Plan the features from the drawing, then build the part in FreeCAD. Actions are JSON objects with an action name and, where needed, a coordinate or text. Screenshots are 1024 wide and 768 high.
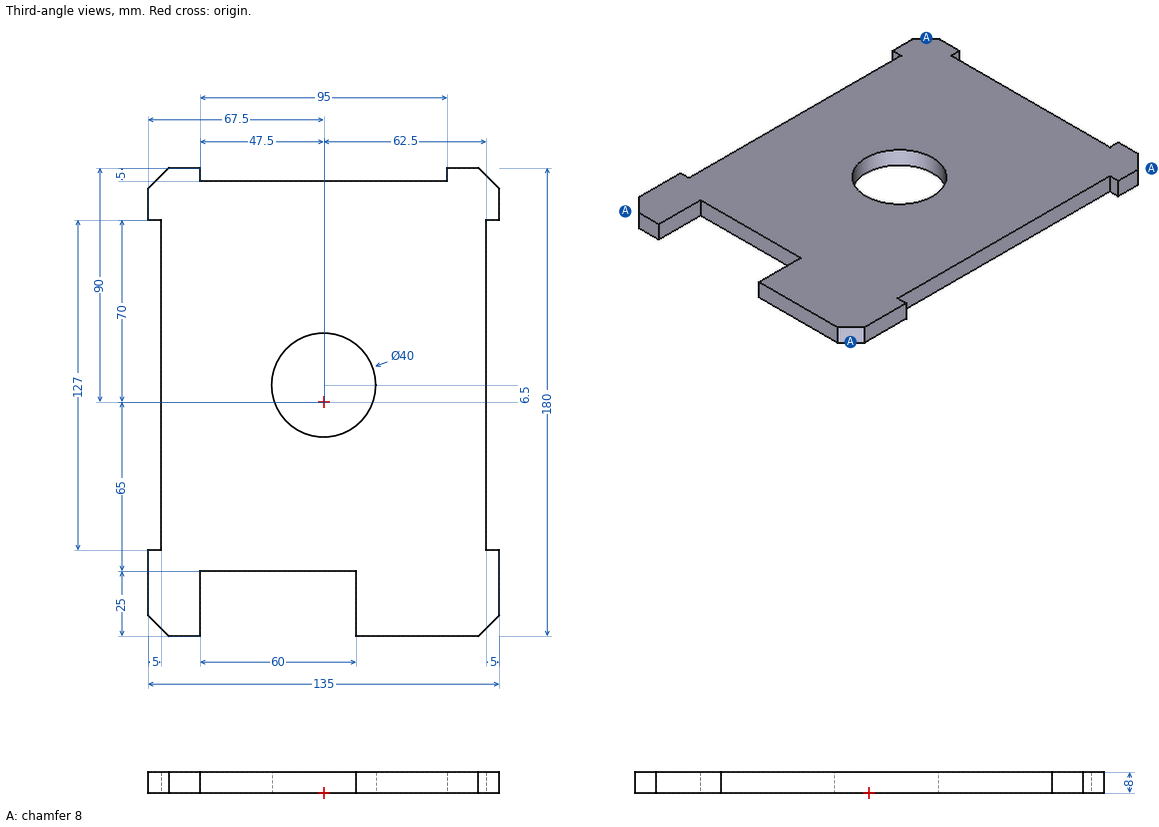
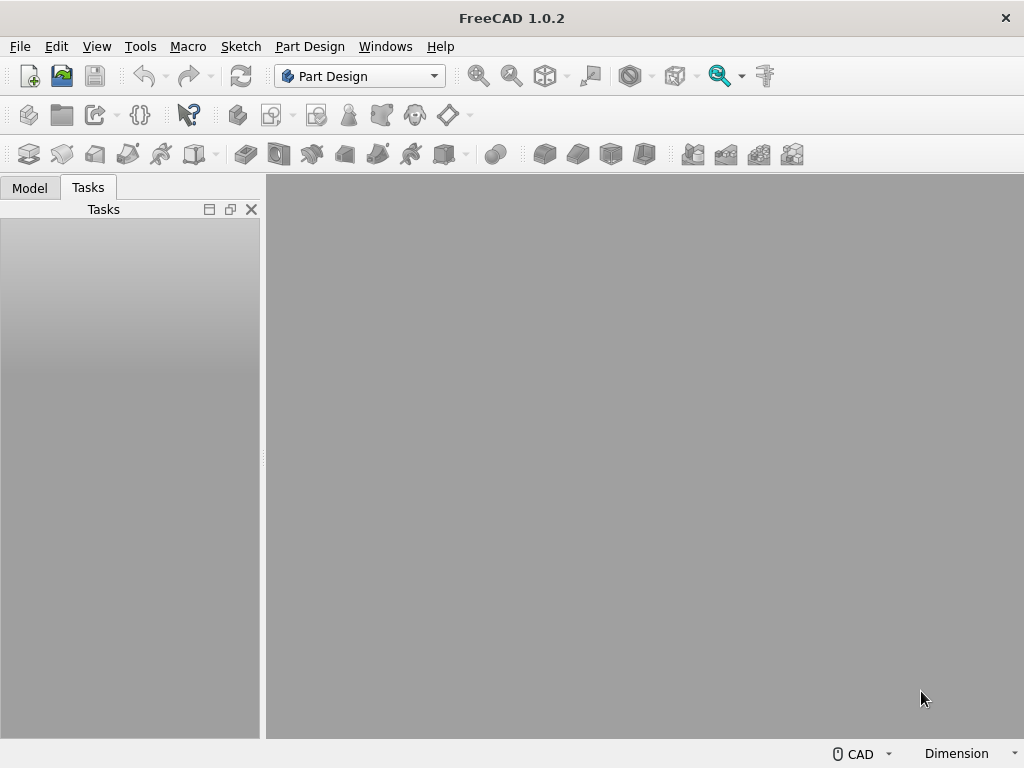
{"action": "left_click", "coordinate": [29, 76]}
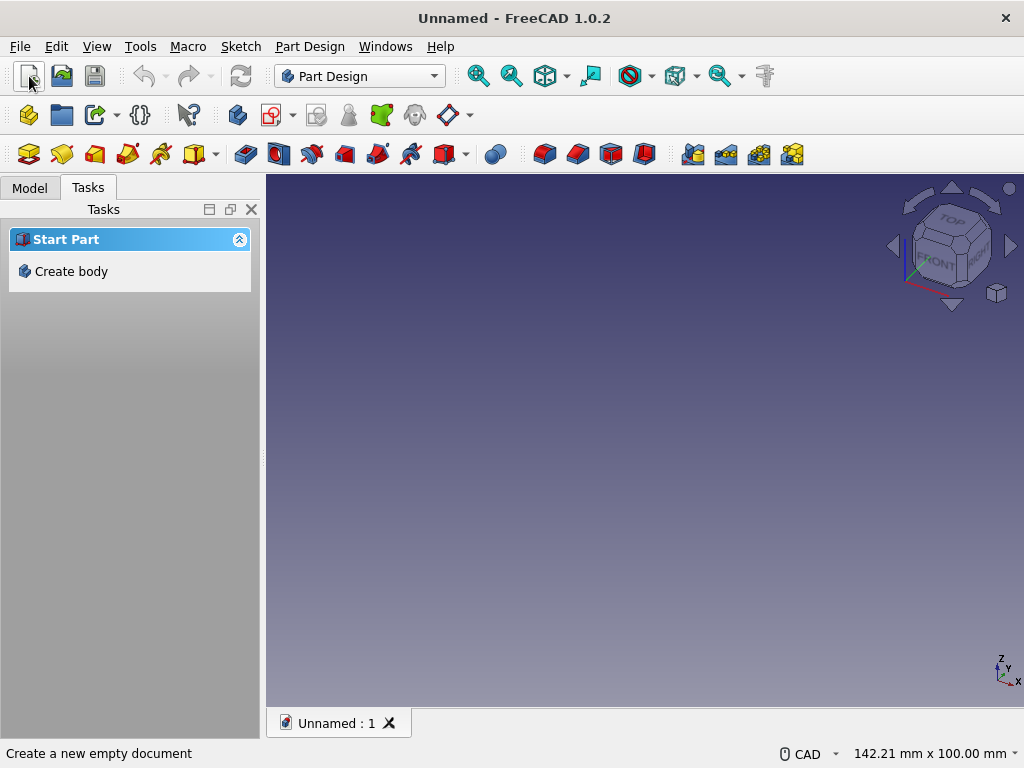
{"action": "left_click", "coordinate": [270, 116]}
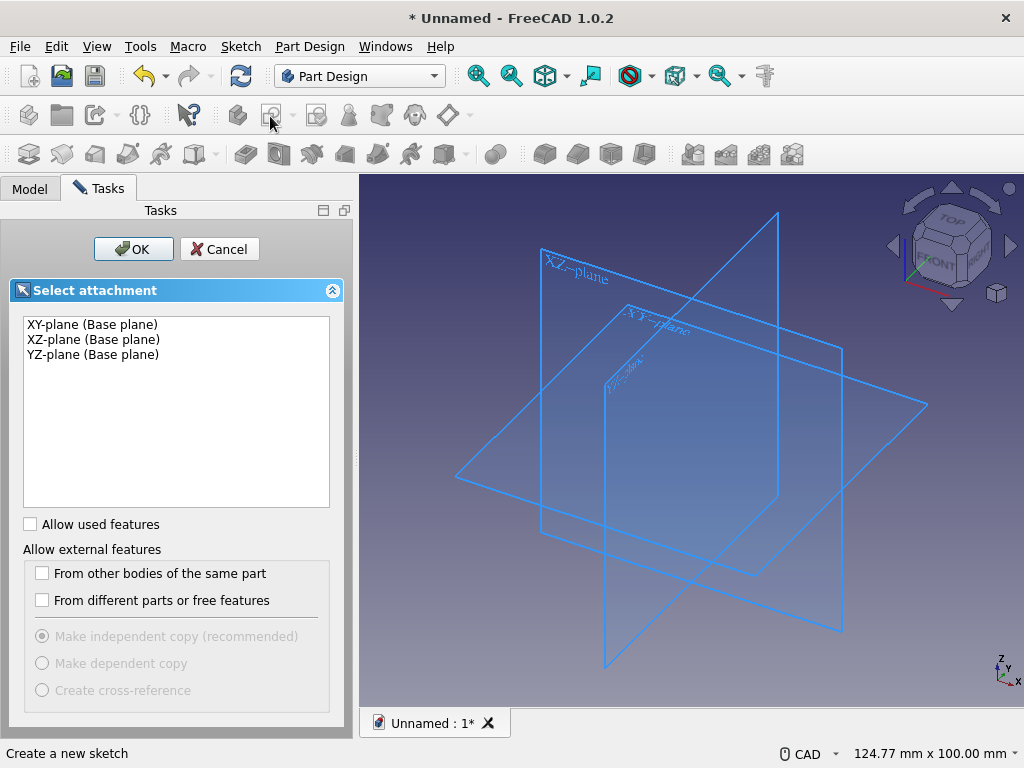
{"action": "left_click", "coordinate": [84, 324]}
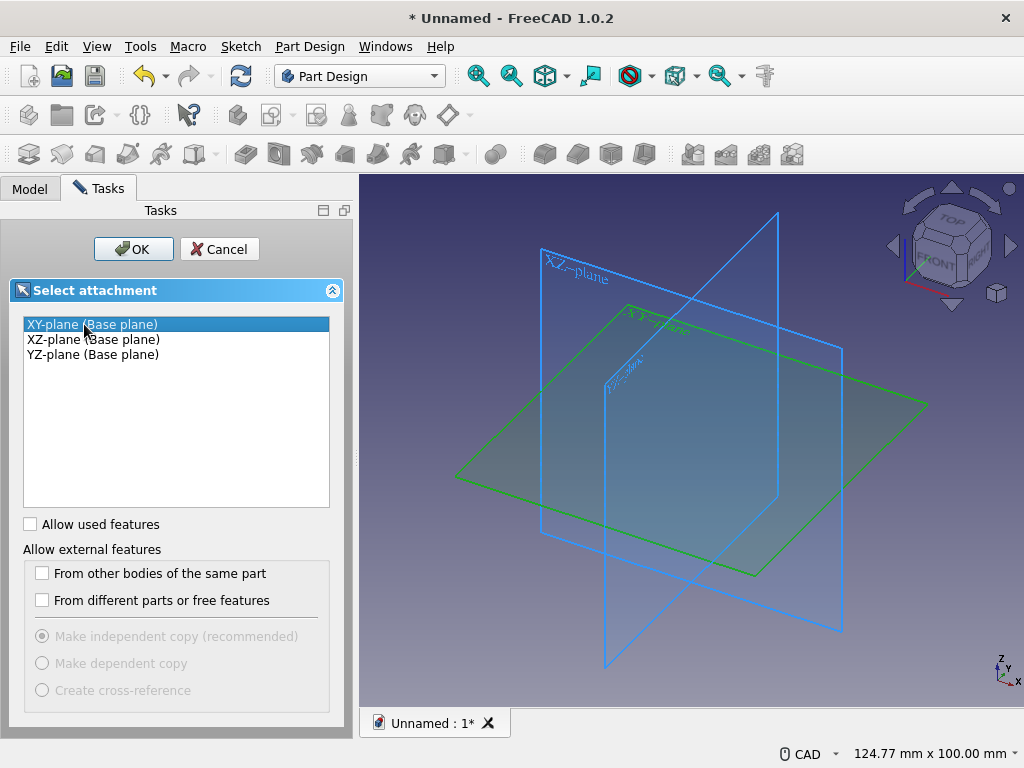
{"action": "left_click", "coordinate": [134, 249]}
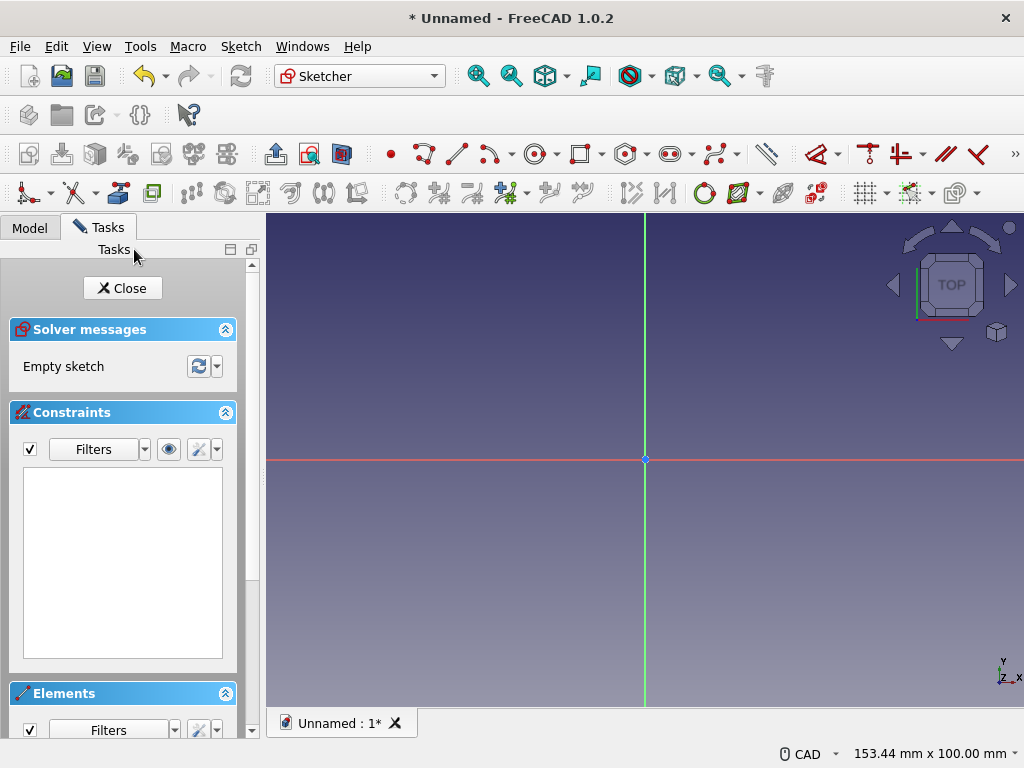
{"action": "scroll", "coordinate": [537, 460], "scroll_direction": "down", "scroll_amount": 5}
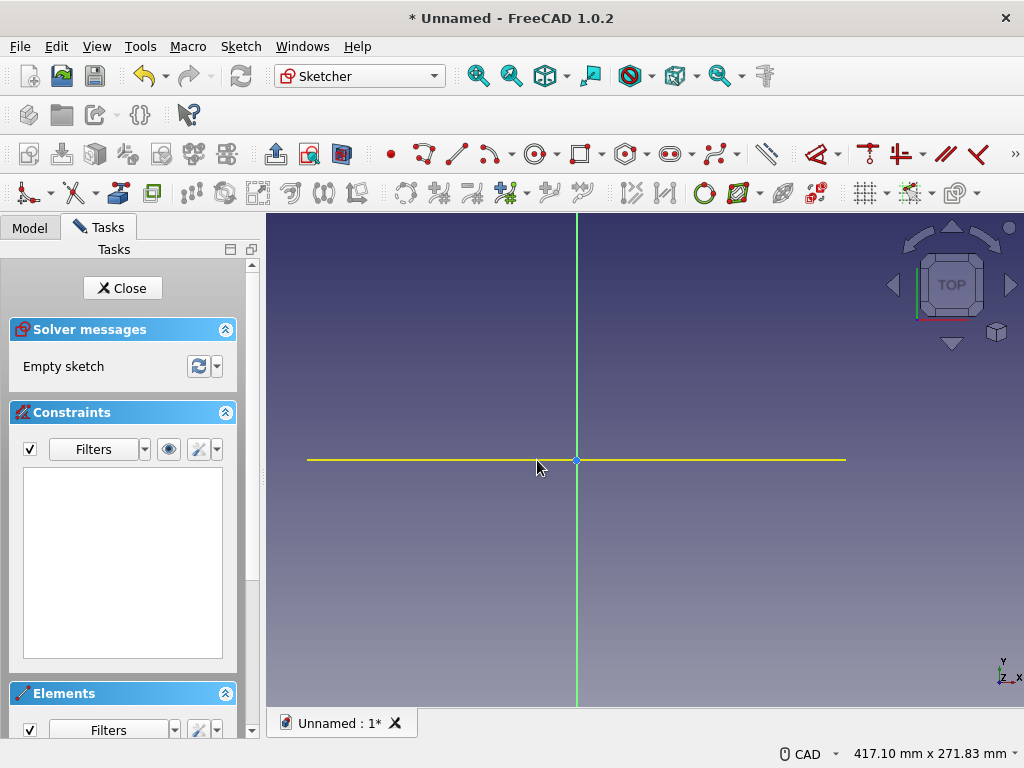
{"action": "key", "text": "g v"}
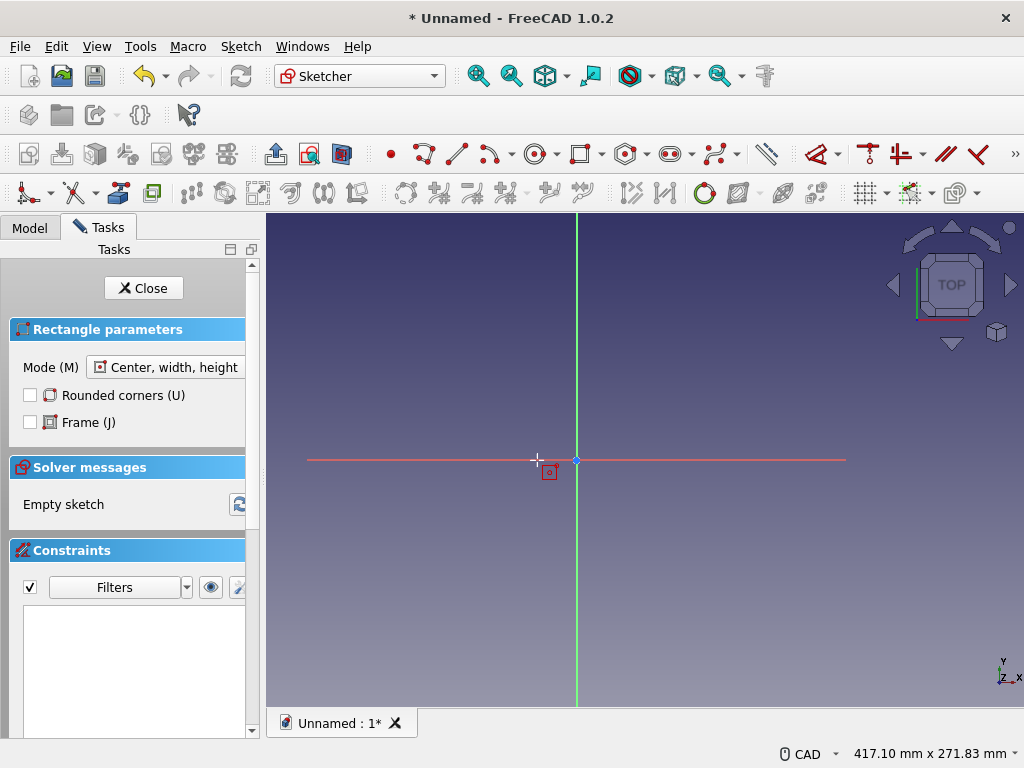
{"action": "left_click", "coordinate": [577, 460]}
{"action": "left_click", "coordinate": [700, 297]}
{"action": "key", "text": "Escape"}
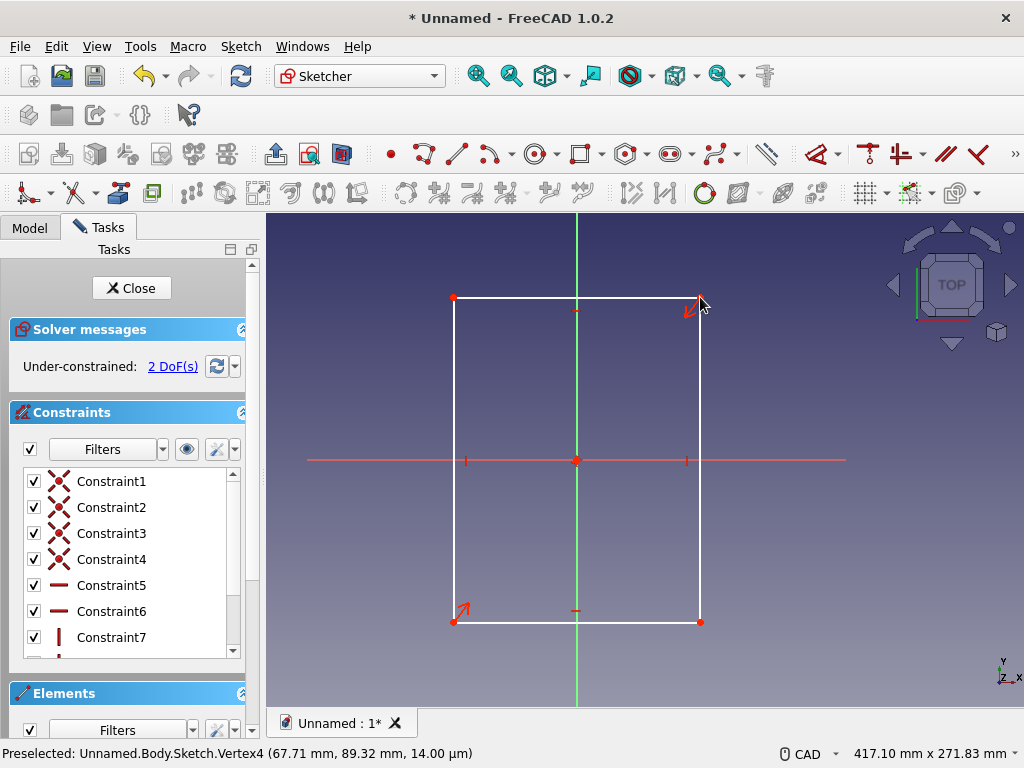
{"action": "left_click", "coordinate": [528, 623]}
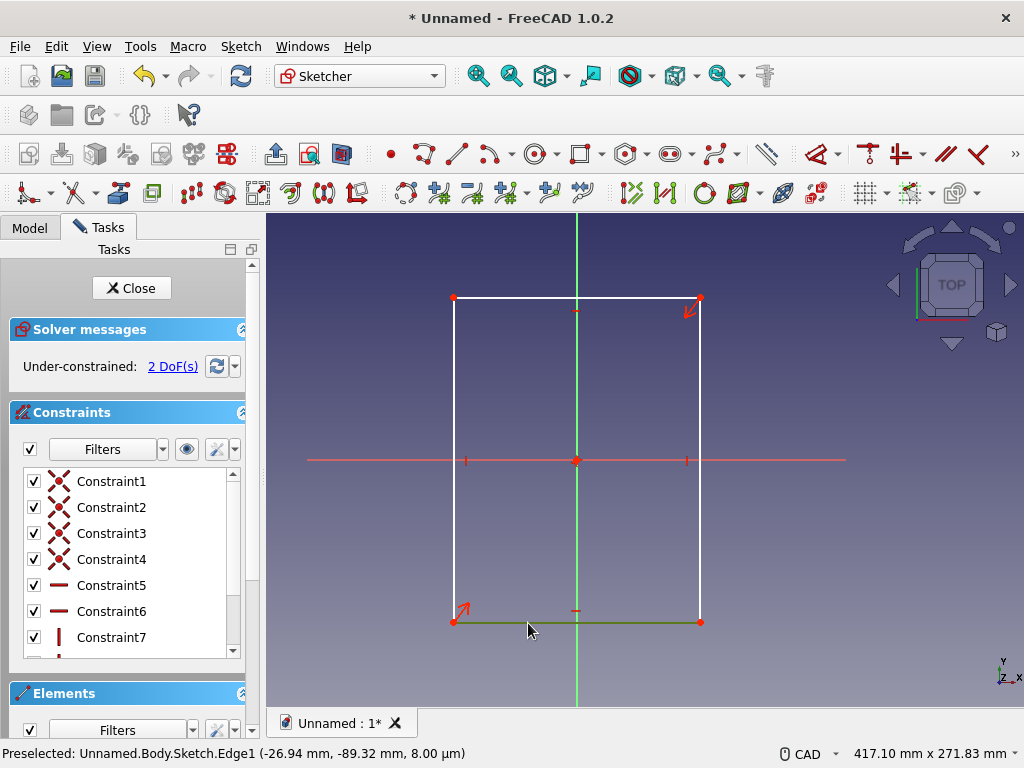
{"action": "key", "text": "l"}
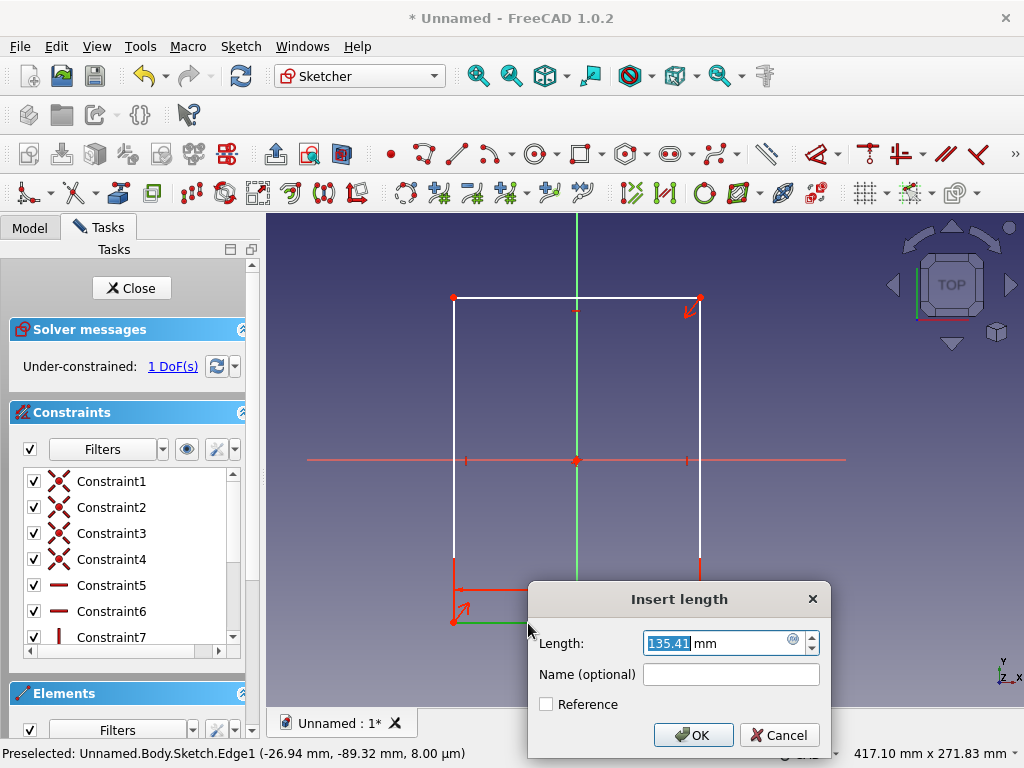
{"action": "type", "text": "135"}
{"action": "key", "text": "Return"}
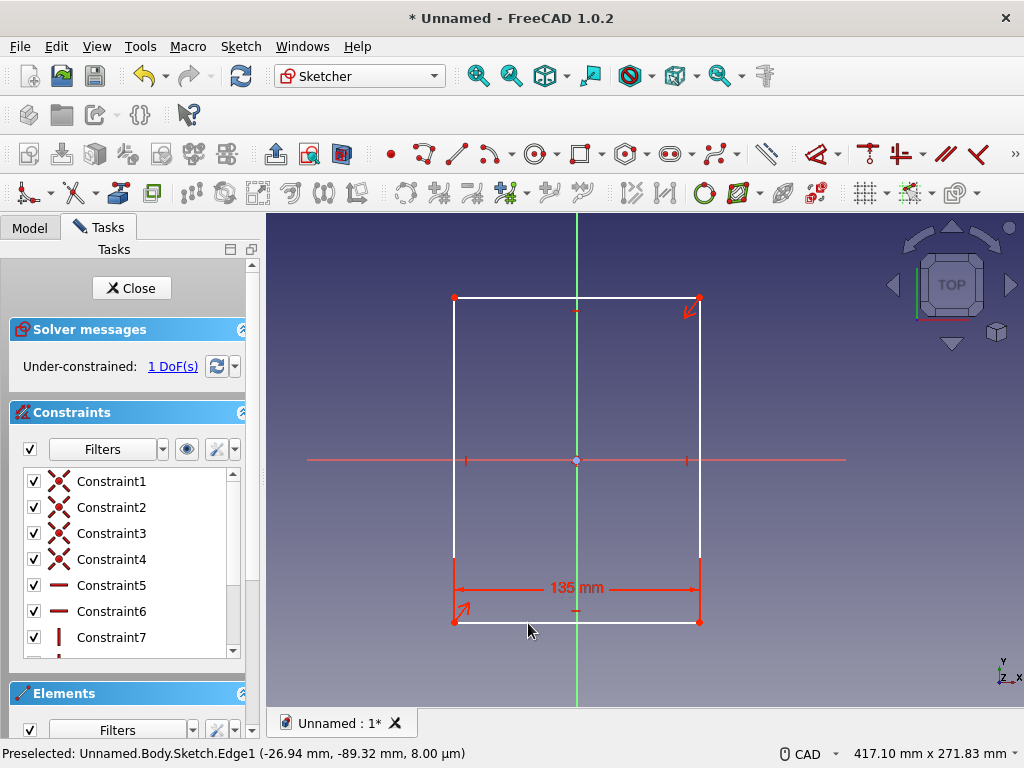
{"action": "left_click", "coordinate": [700, 525]}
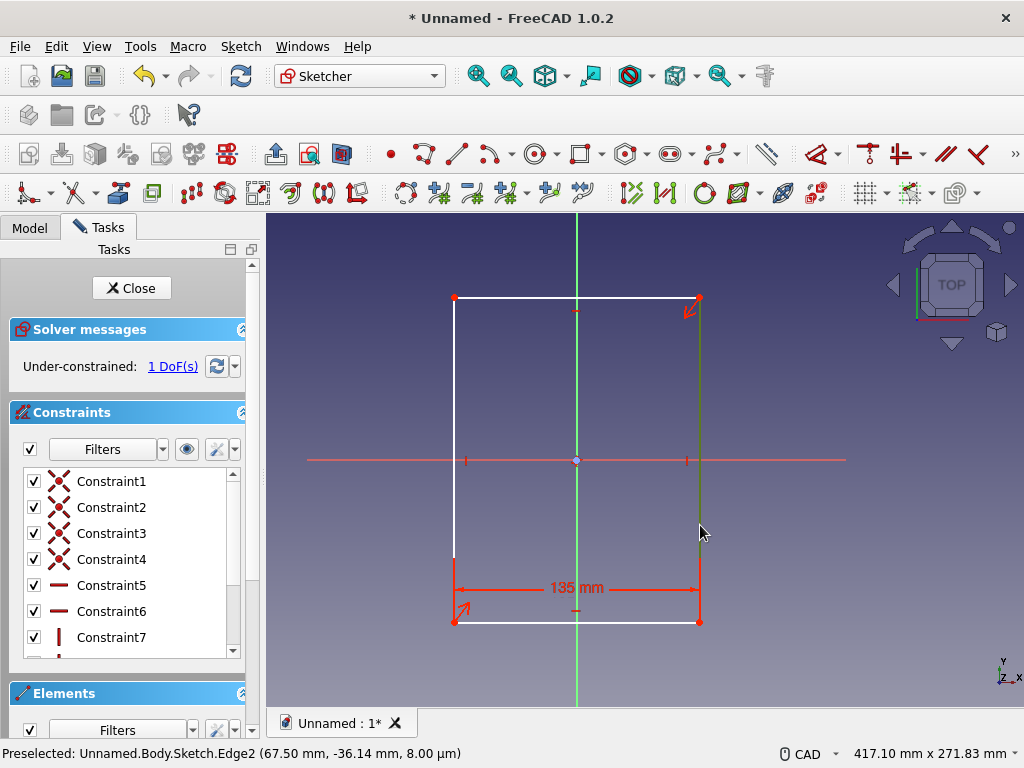
{"action": "key", "text": "i"}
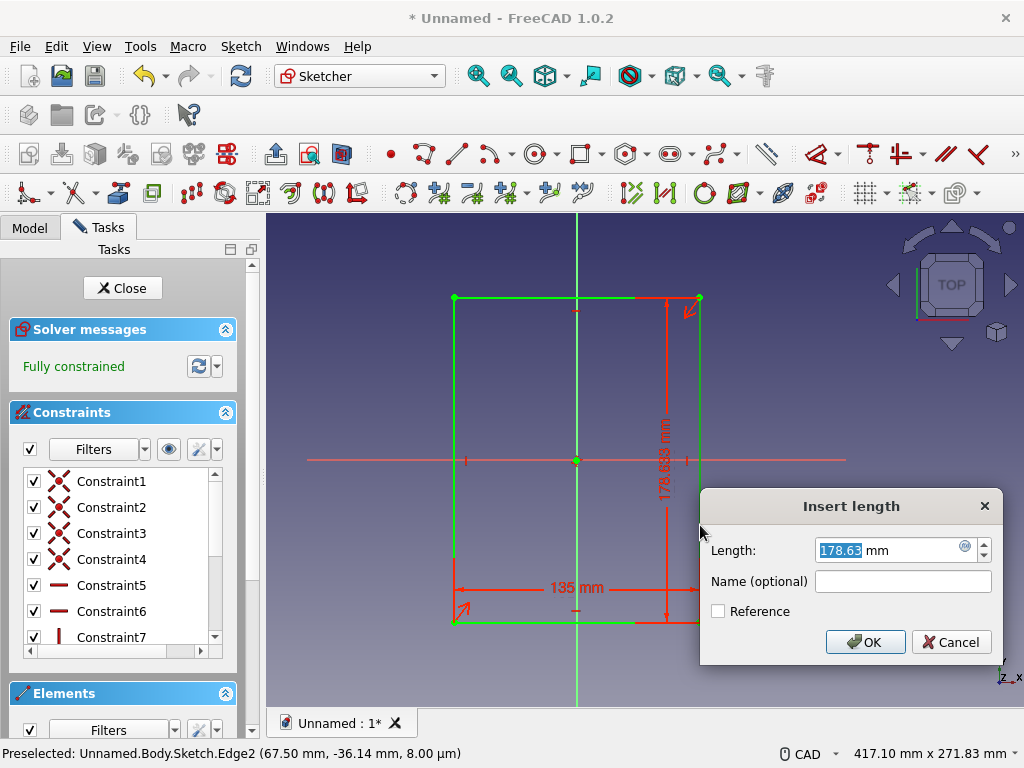
{"action": "type", "text": "180"}
{"action": "key", "text": "Return"}